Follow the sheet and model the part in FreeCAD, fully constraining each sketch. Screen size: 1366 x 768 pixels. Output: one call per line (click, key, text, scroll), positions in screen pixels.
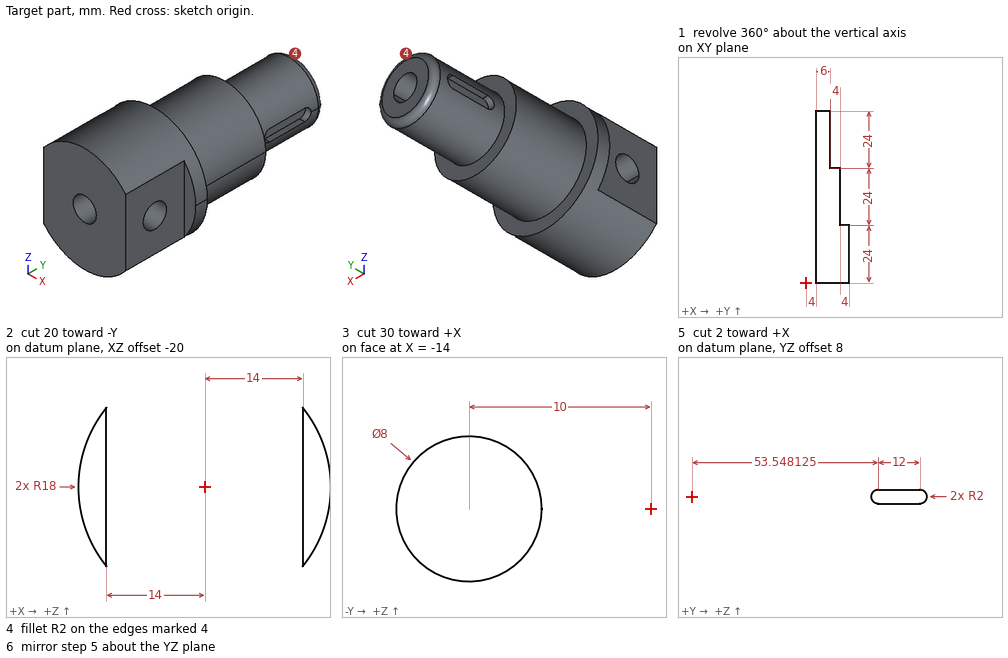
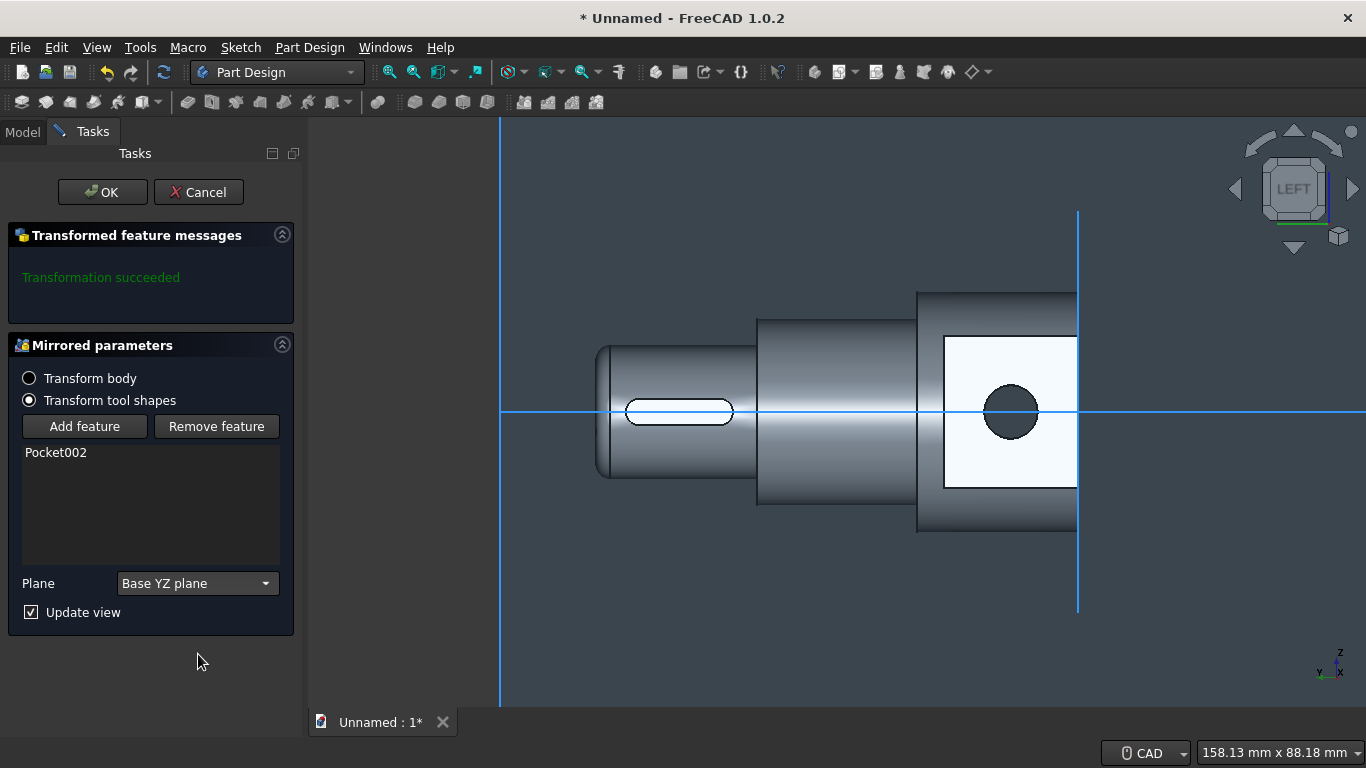
click(103, 192)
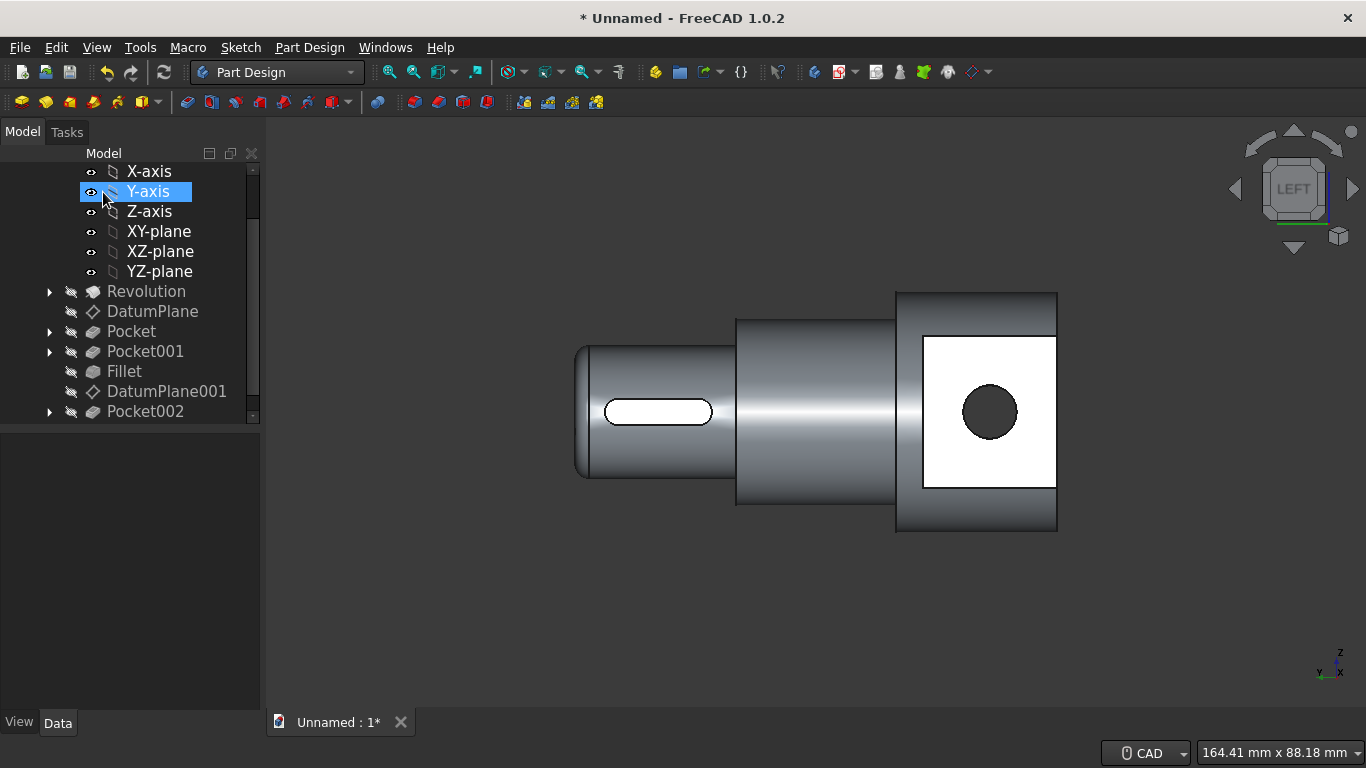
key(0)